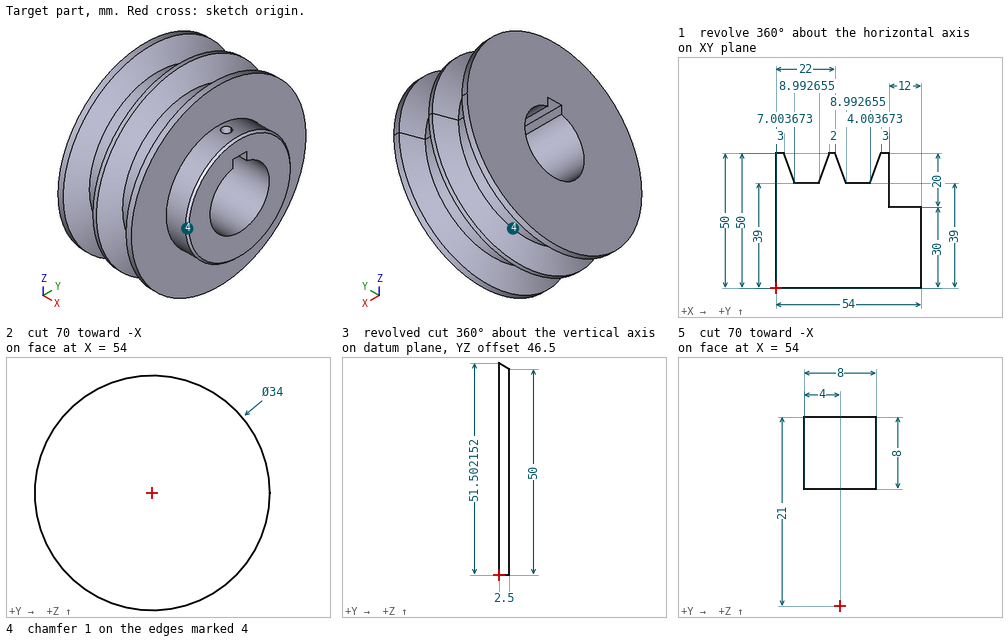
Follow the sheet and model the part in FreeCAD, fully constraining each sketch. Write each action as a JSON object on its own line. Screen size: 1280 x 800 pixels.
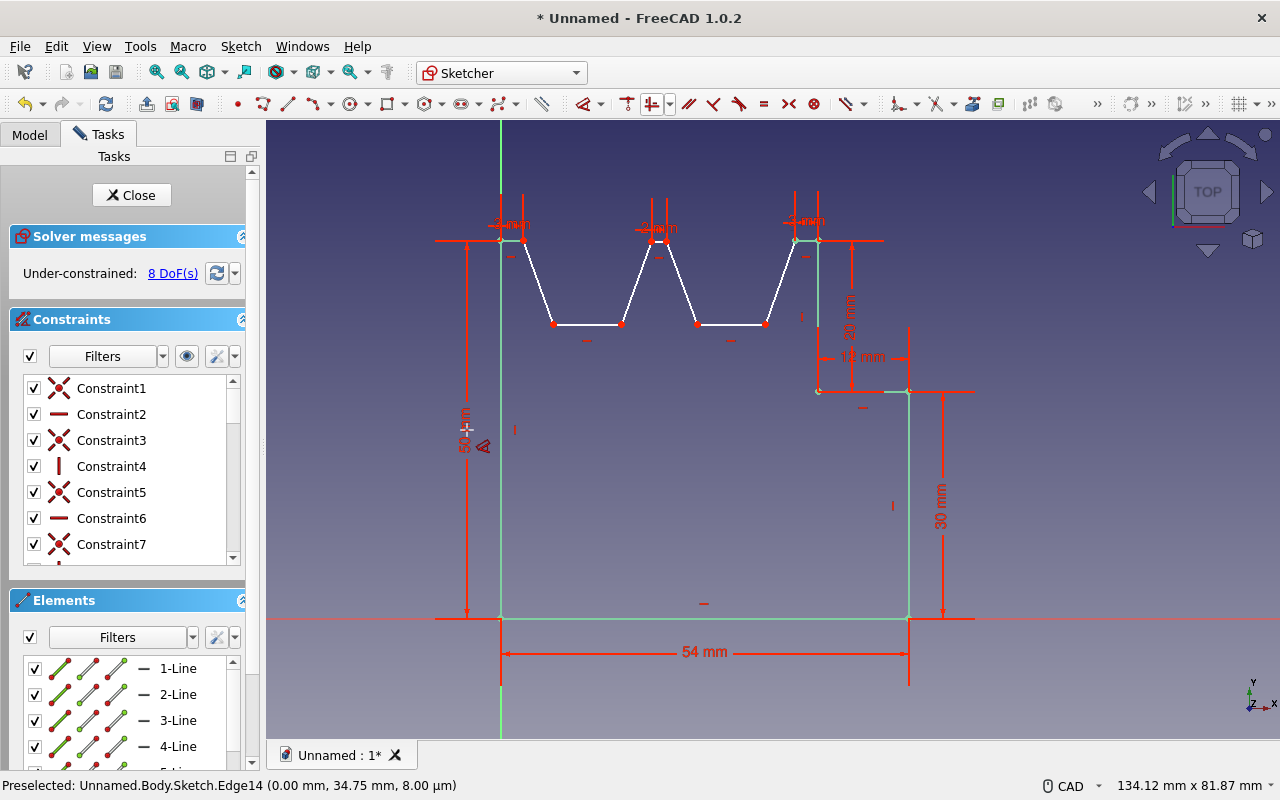
{"action": "left_click", "coordinate": [766, 325]}
{"action": "left_click", "coordinate": [467, 472]}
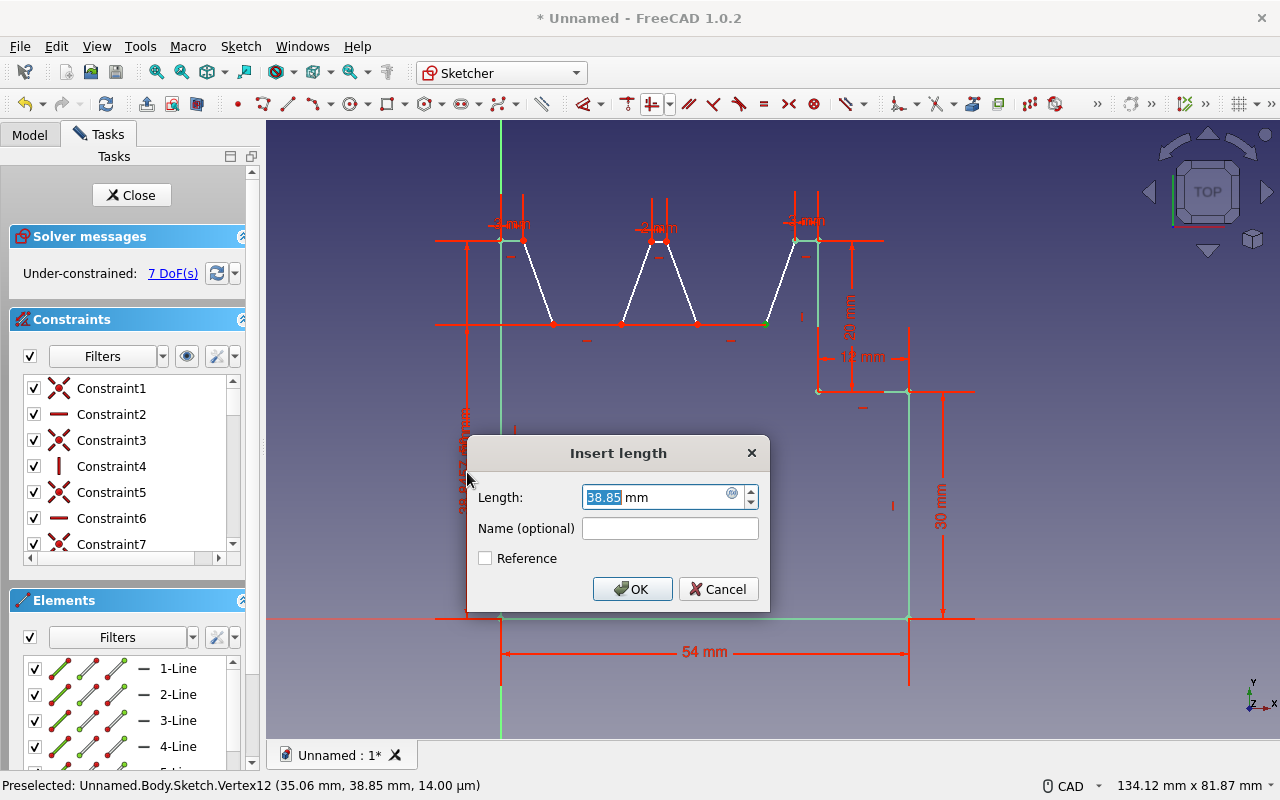
{"action": "type", "text": "39"}
{"action": "key", "text": "Return"}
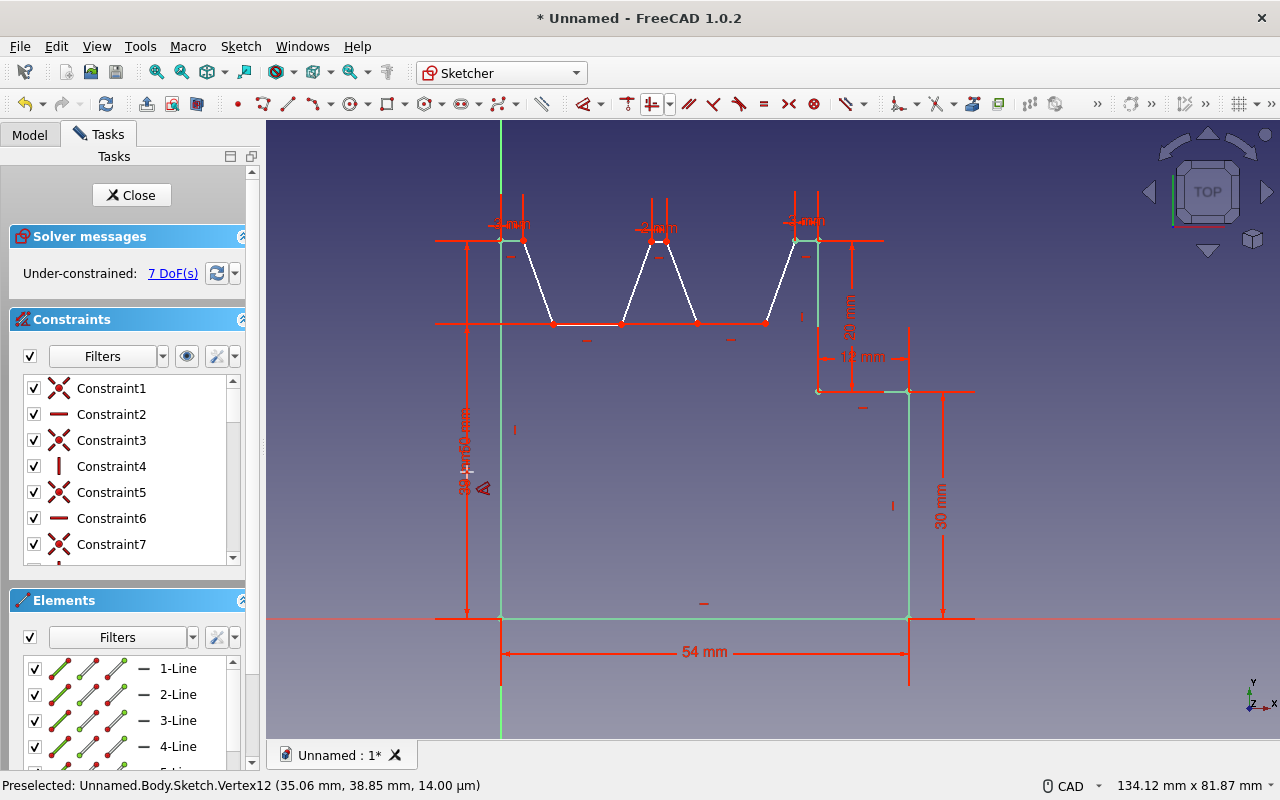
{"action": "left_click", "coordinate": [667, 242]}
{"action": "left_click", "coordinate": [584, 653]}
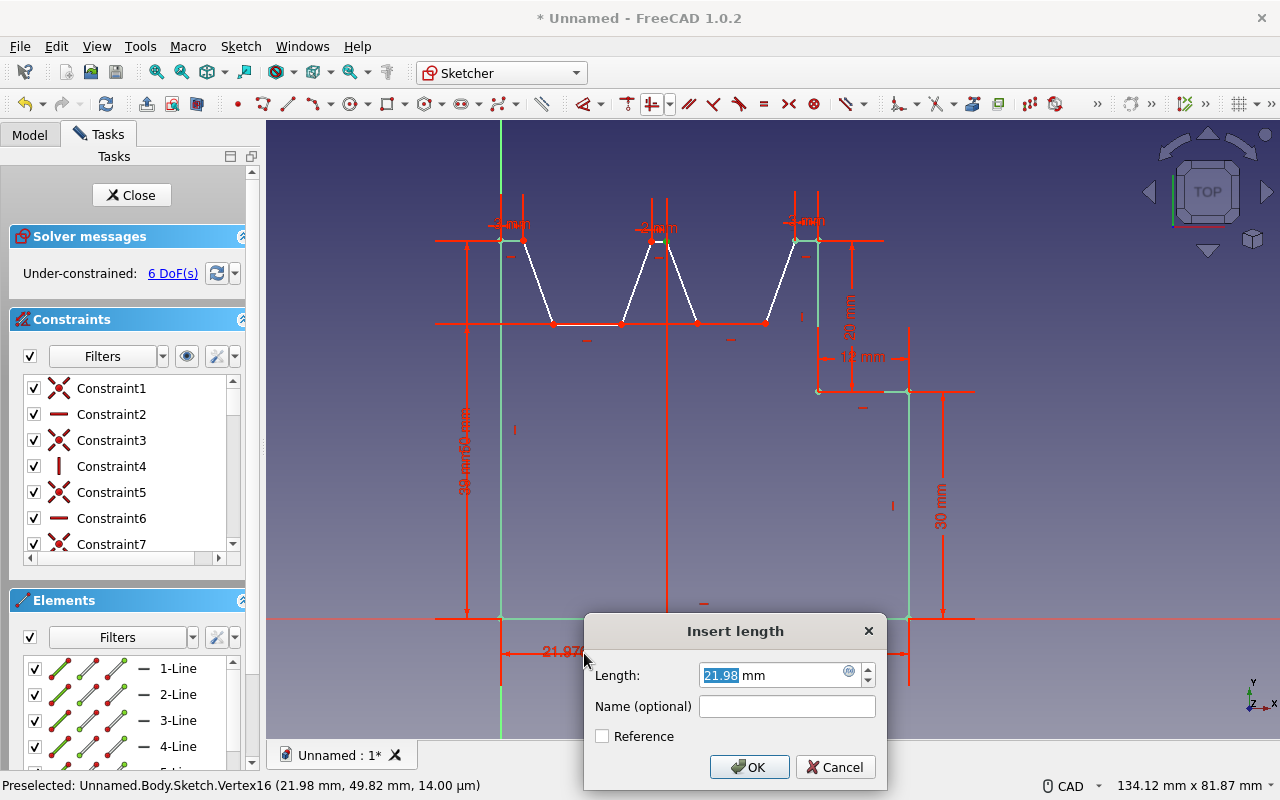
{"action": "type", "text": "22"}
{"action": "key", "text": "Return"}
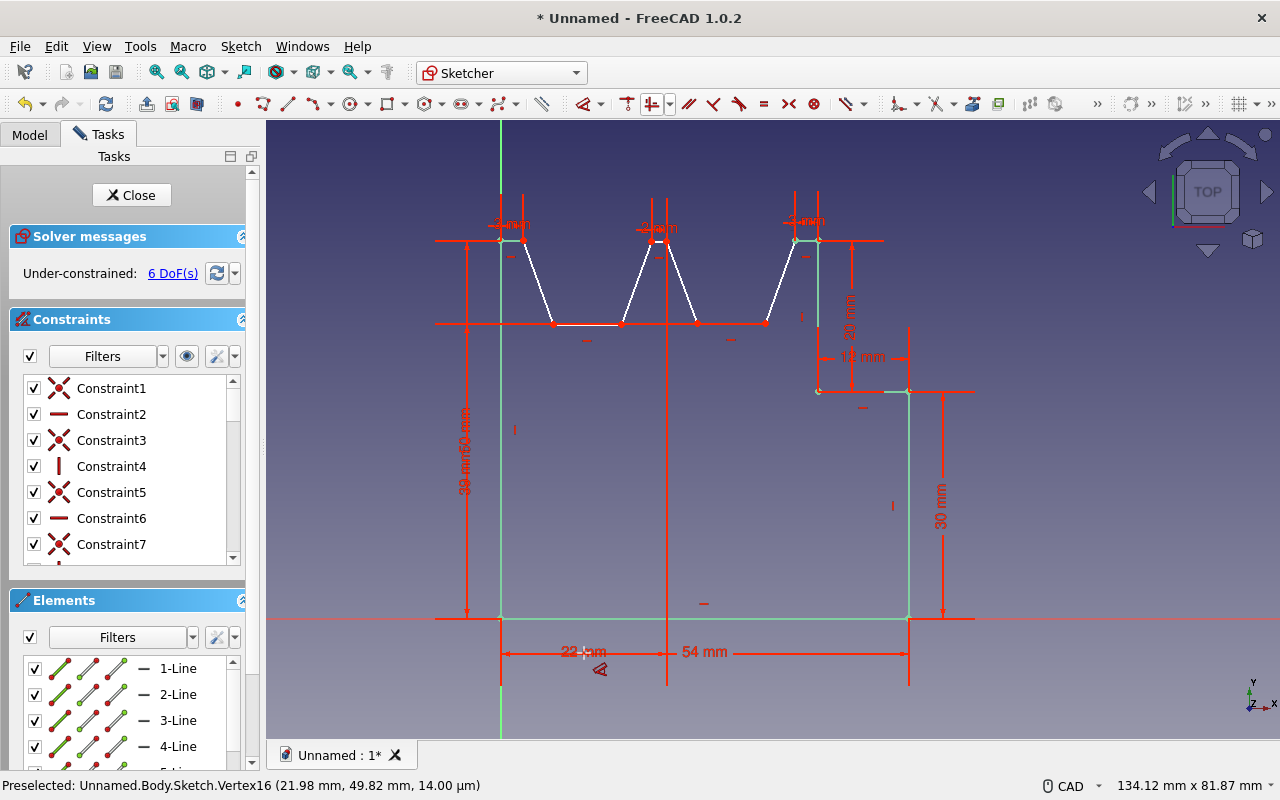
{"action": "left_click", "coordinate": [667, 242]}
{"action": "left_click", "coordinate": [467, 344]}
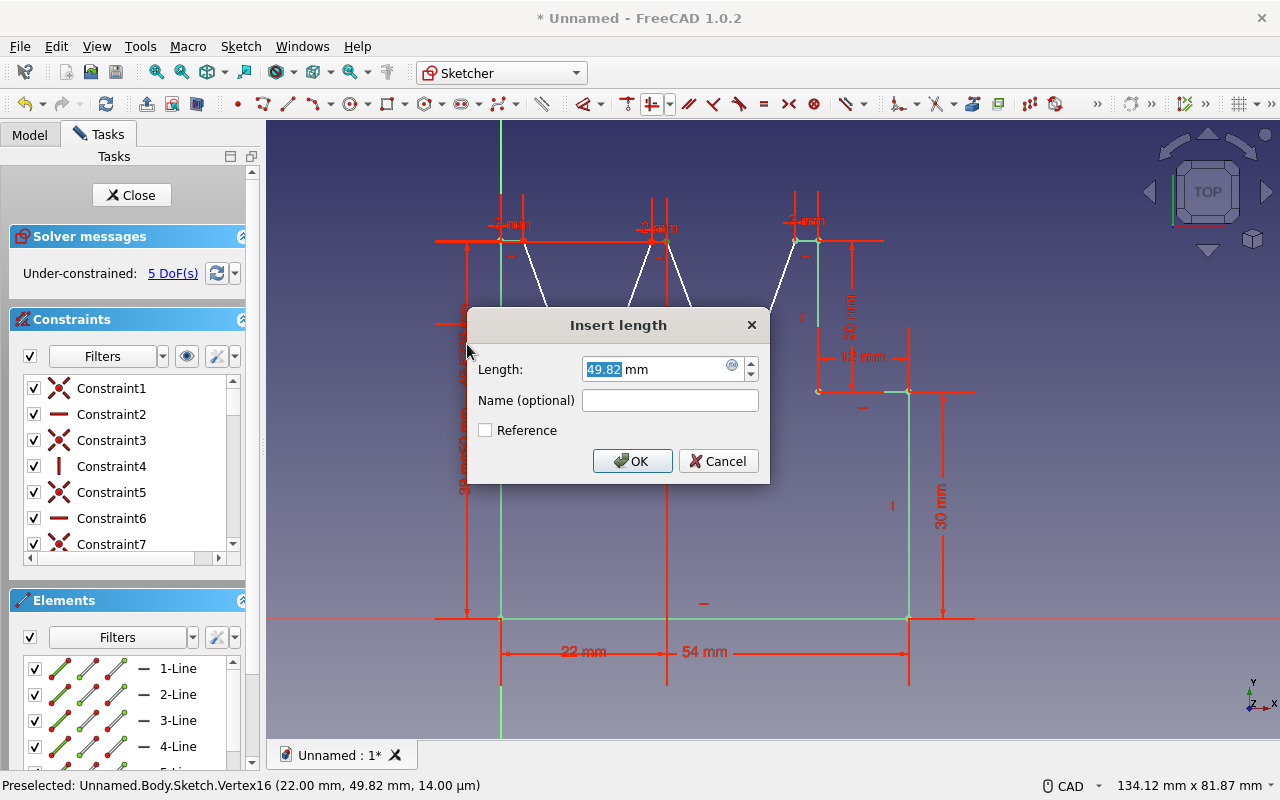
{"action": "type", "text": "50"}
{"action": "key", "text": "Return"}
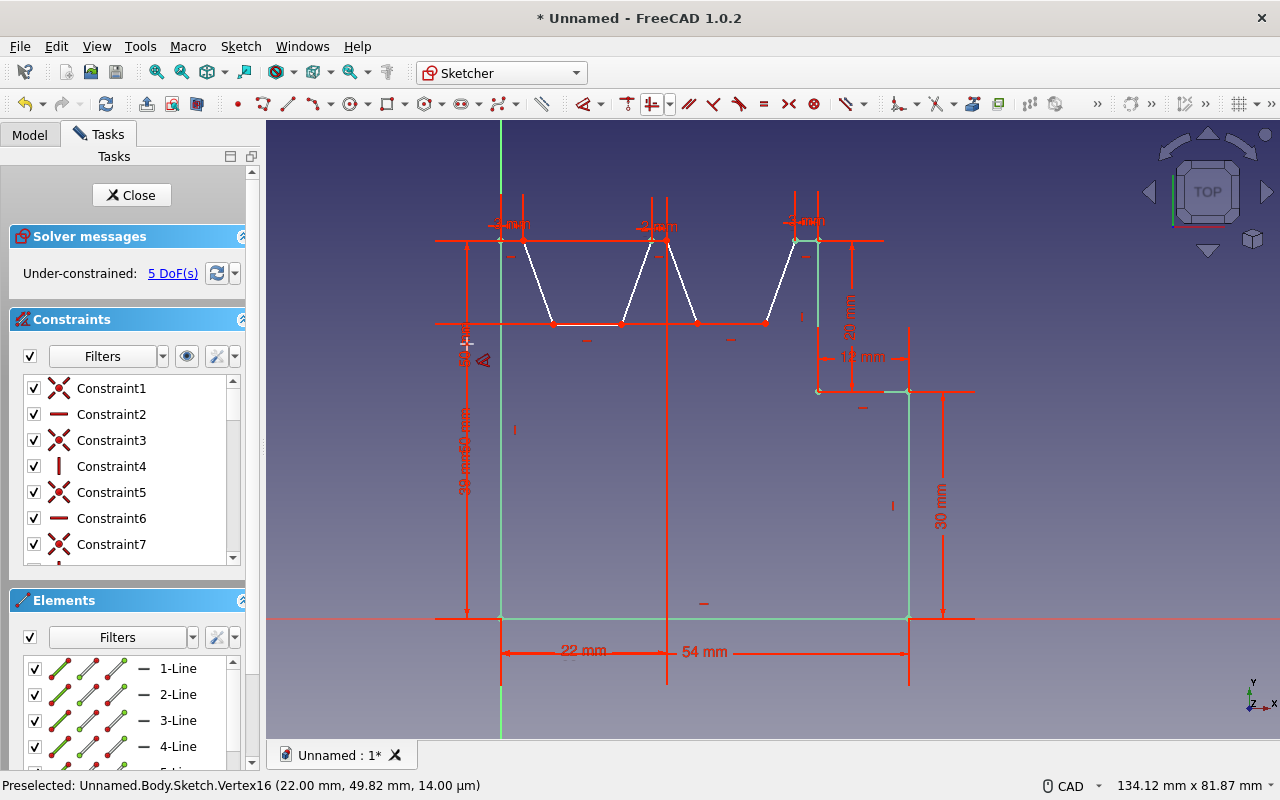
{"action": "left_click", "coordinate": [622, 325]}
{"action": "left_click", "coordinate": [467, 404]}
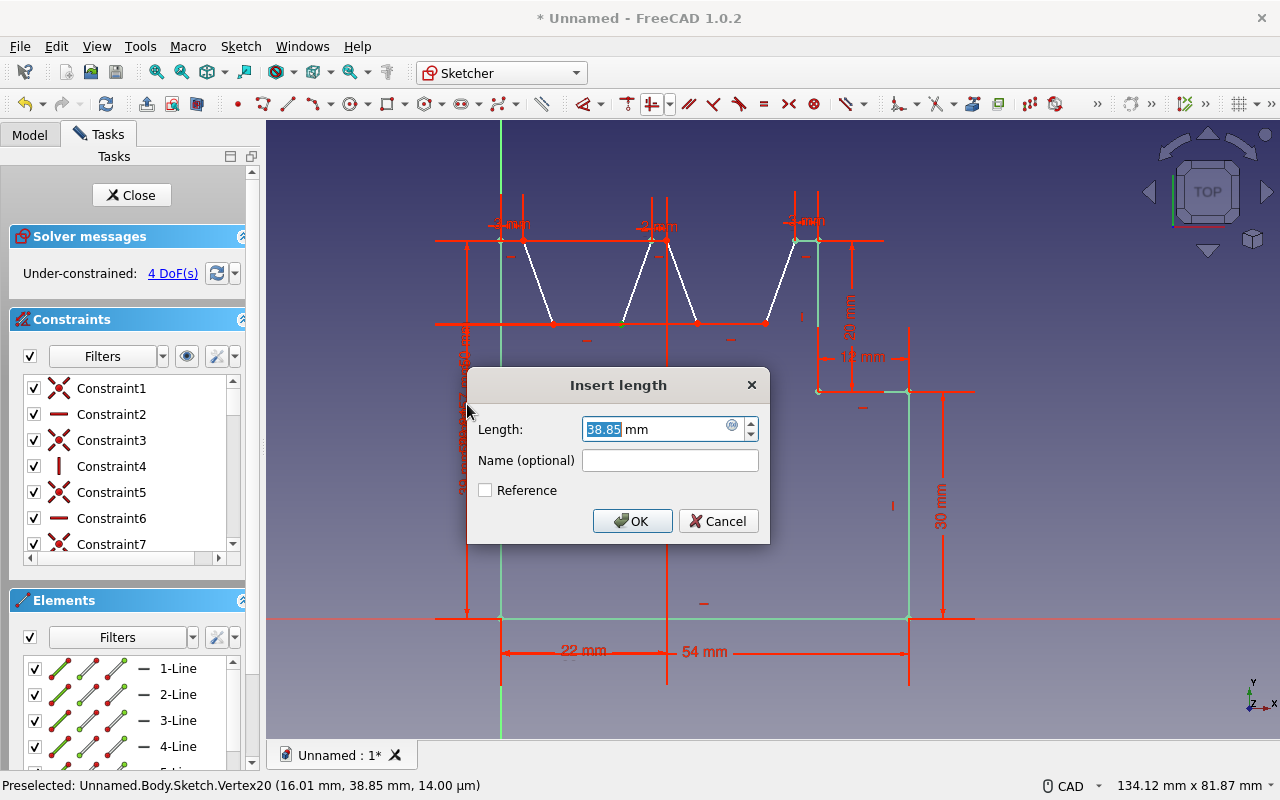
{"action": "type", "text": "39"}
{"action": "key", "text": "Return"}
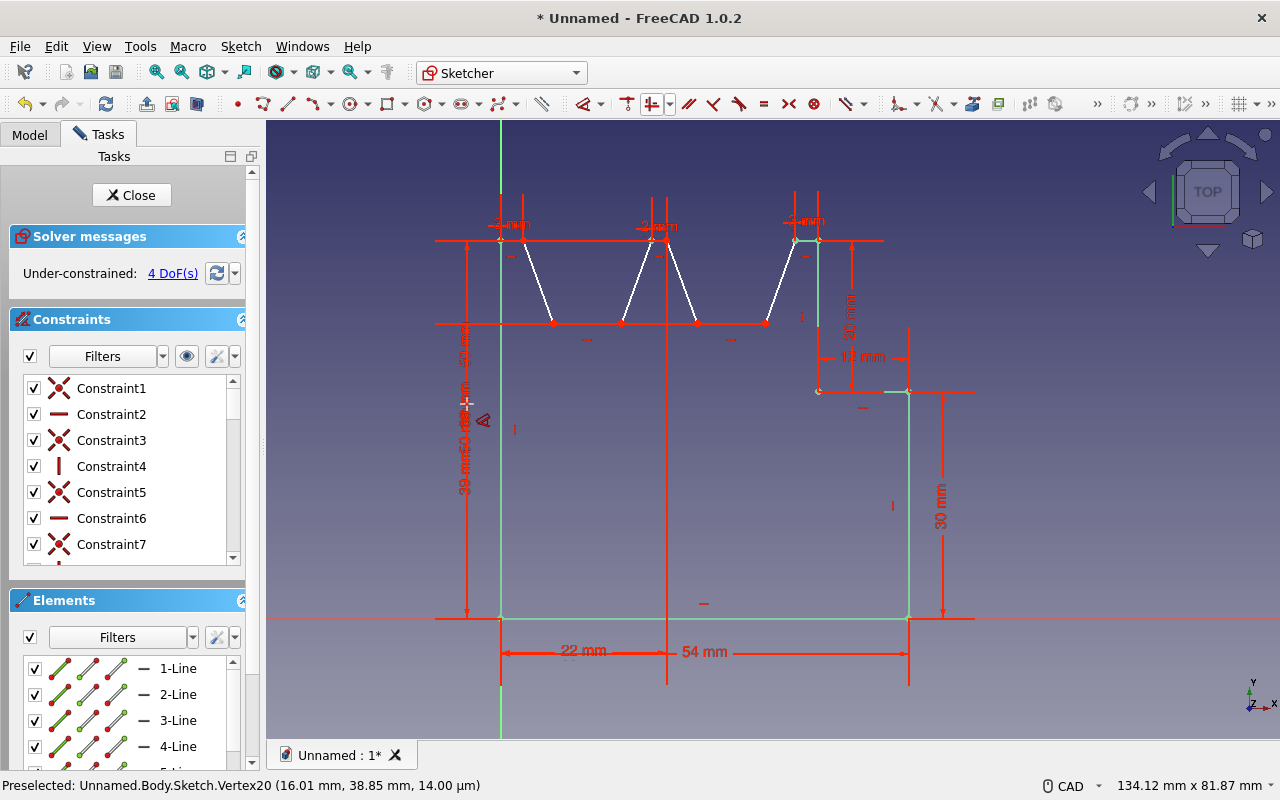
{"action": "left_click", "coordinate": [745, 324]}
{"action": "left_click", "coordinate": [732, 290]}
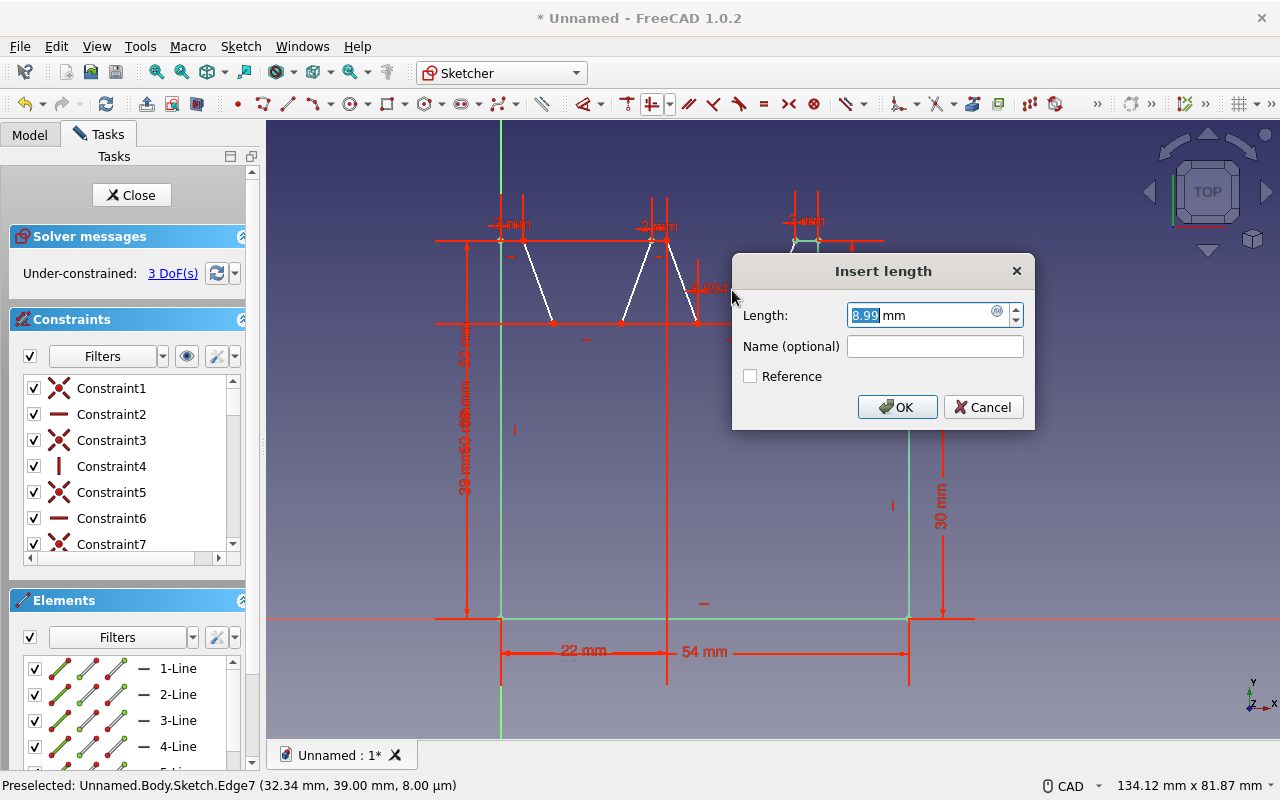
{"action": "type", "text": "8.992655"}
{"action": "key", "text": "Return"}